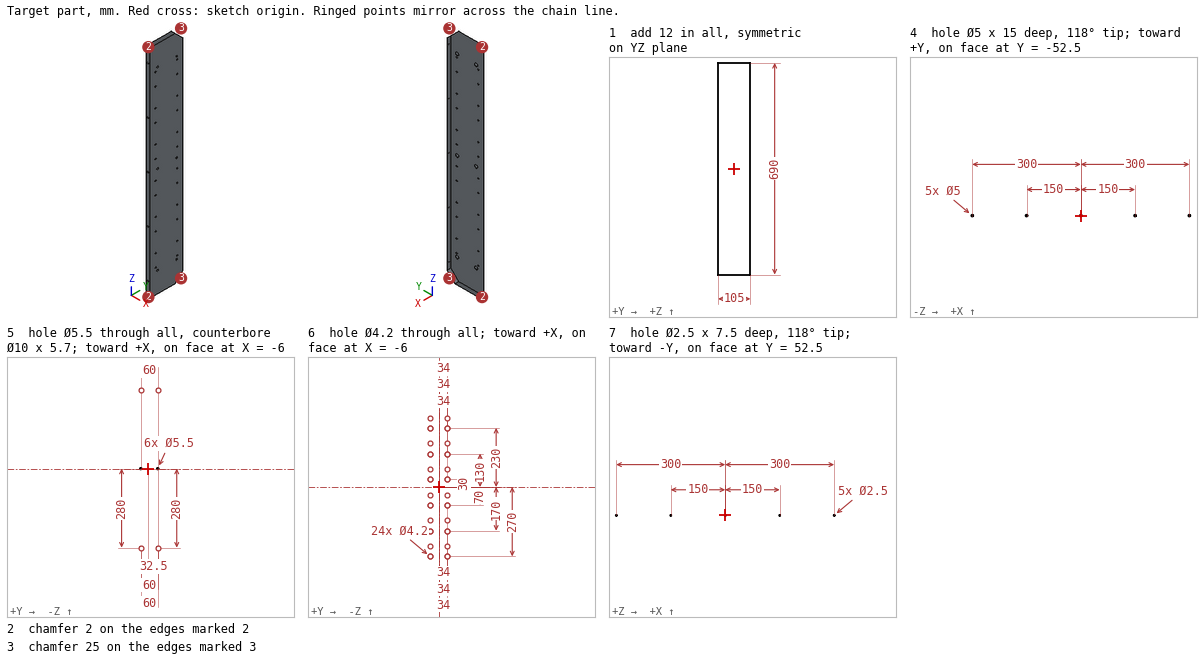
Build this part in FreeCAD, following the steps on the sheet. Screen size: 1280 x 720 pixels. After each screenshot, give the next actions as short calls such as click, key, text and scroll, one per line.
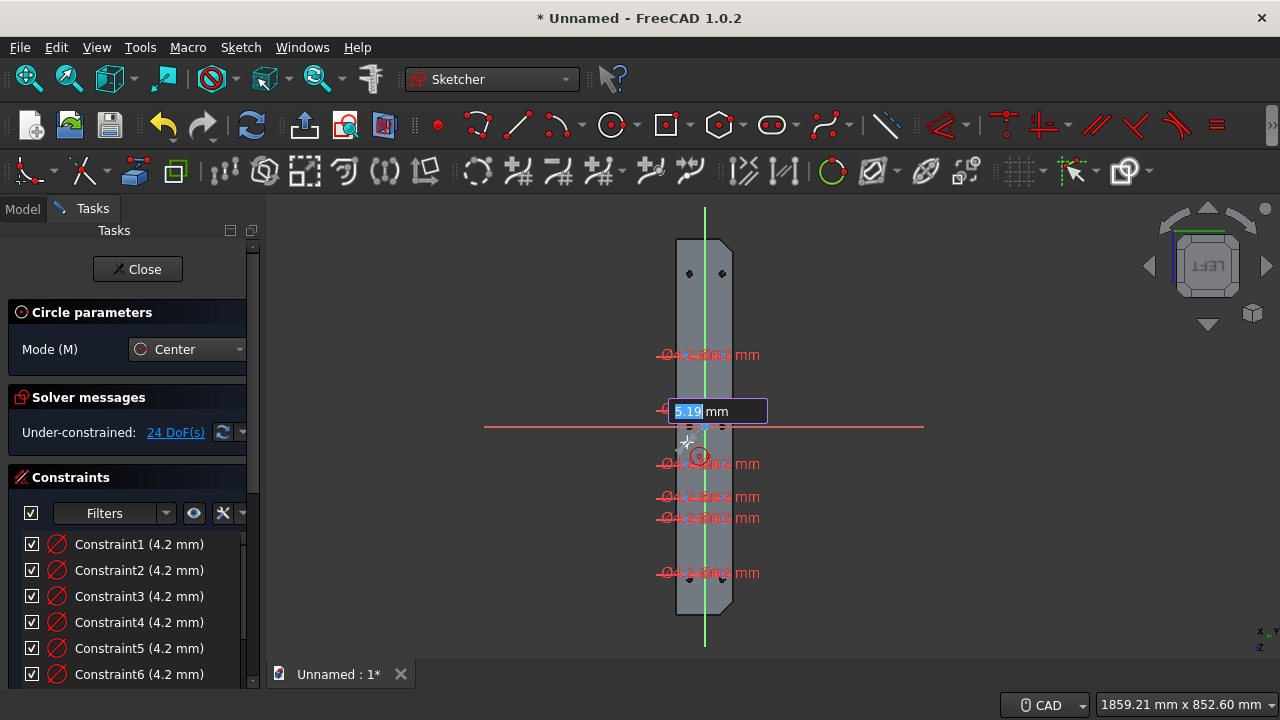
text(4.2)
key(Return)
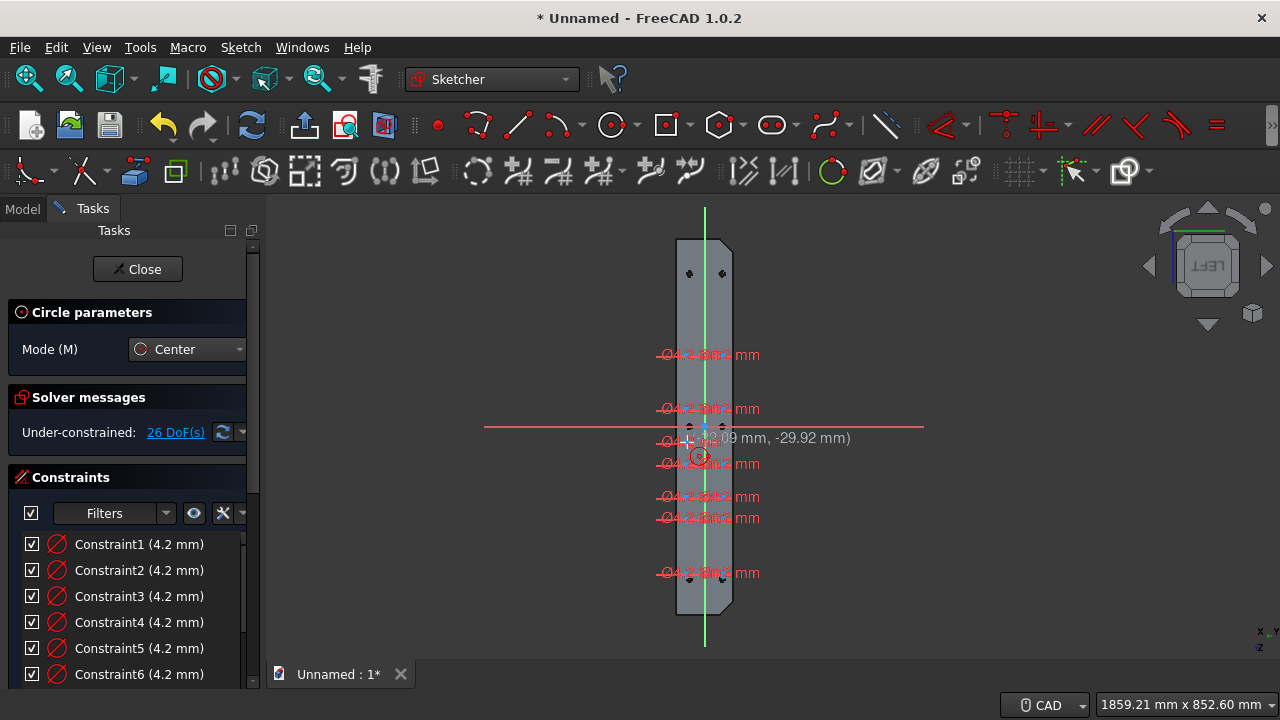
scroll(723, 443, up, 15)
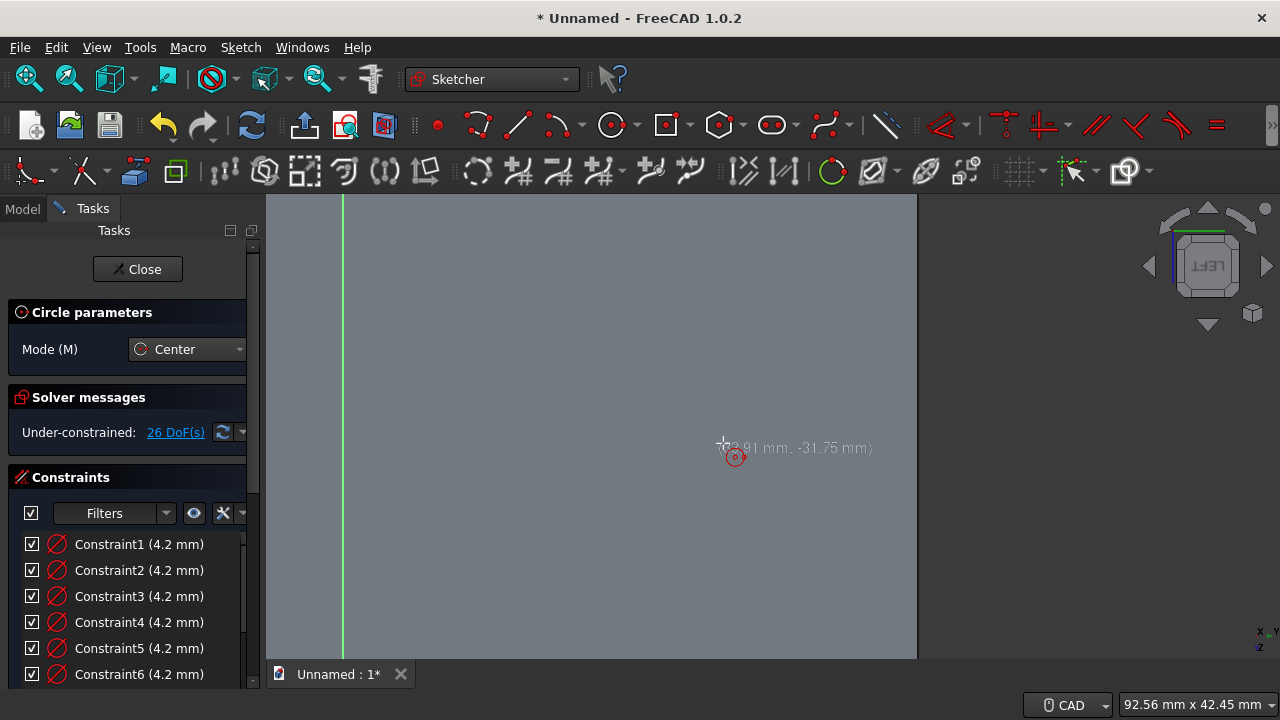
scroll(723, 443, down, 15)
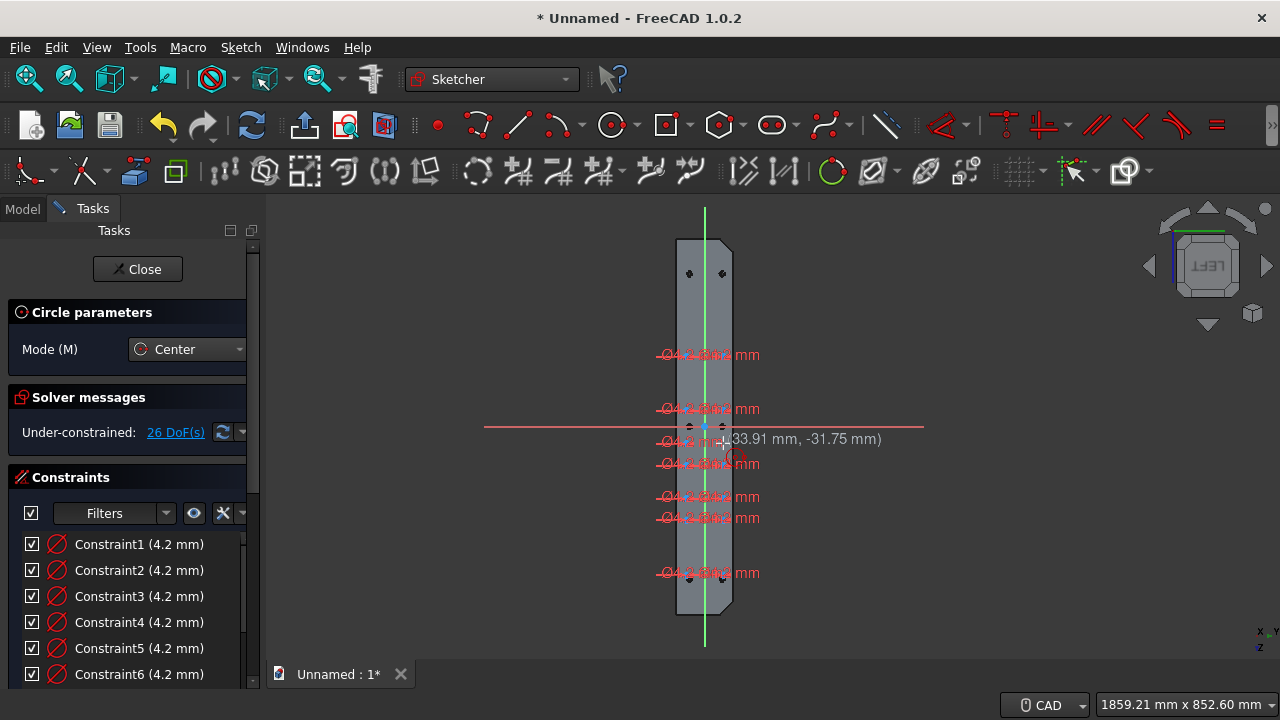
click(723, 443)
move(724, 442)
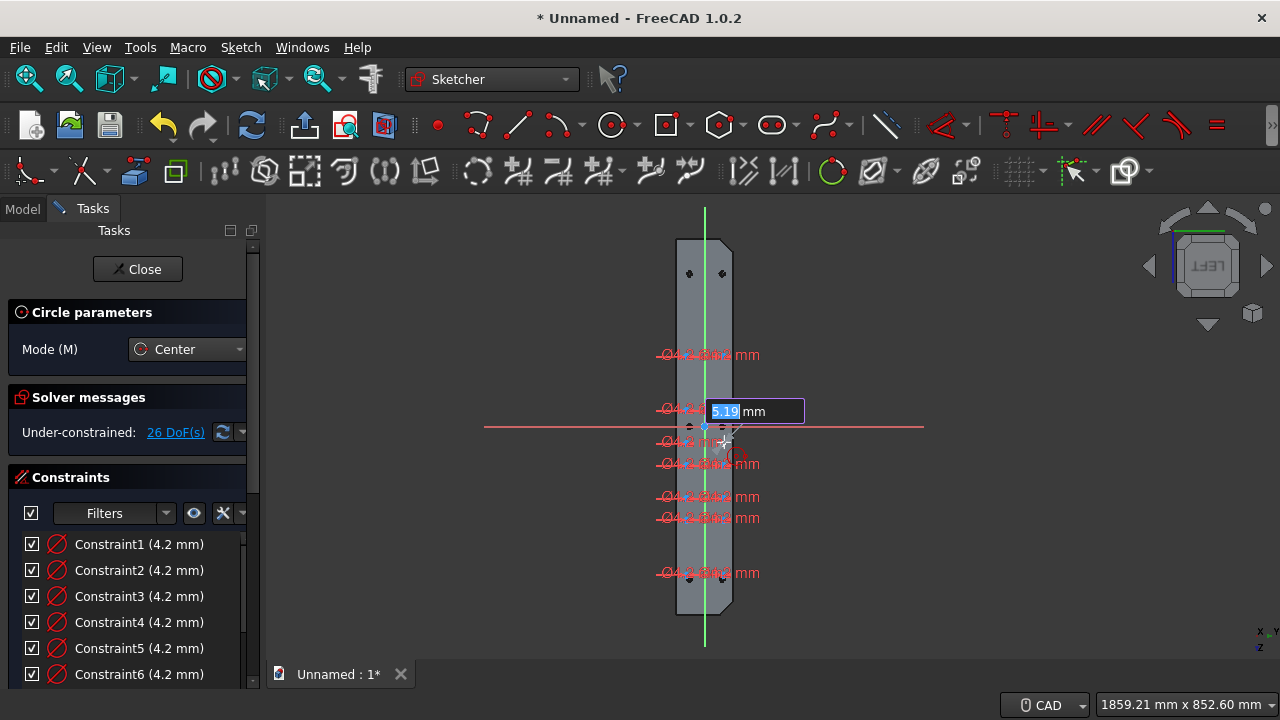
text(4.2)
key(Return)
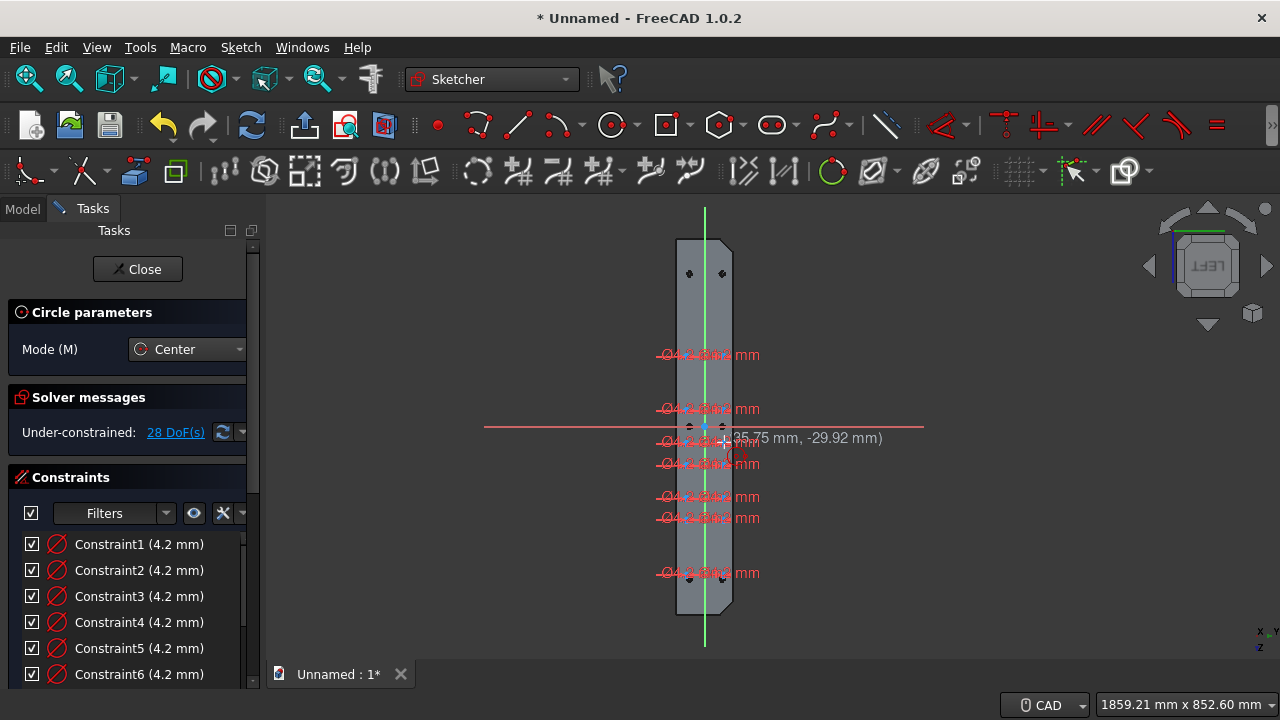
scroll(686, 389, up, 15)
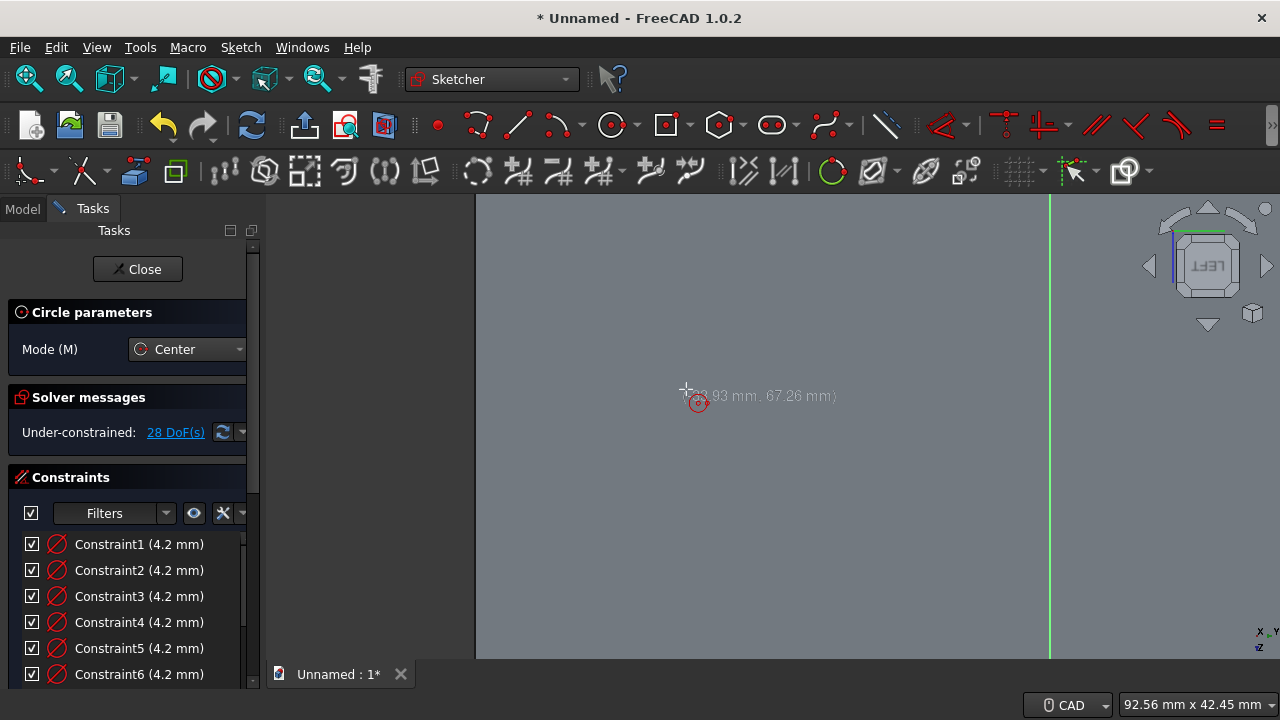
scroll(686, 389, down, 15)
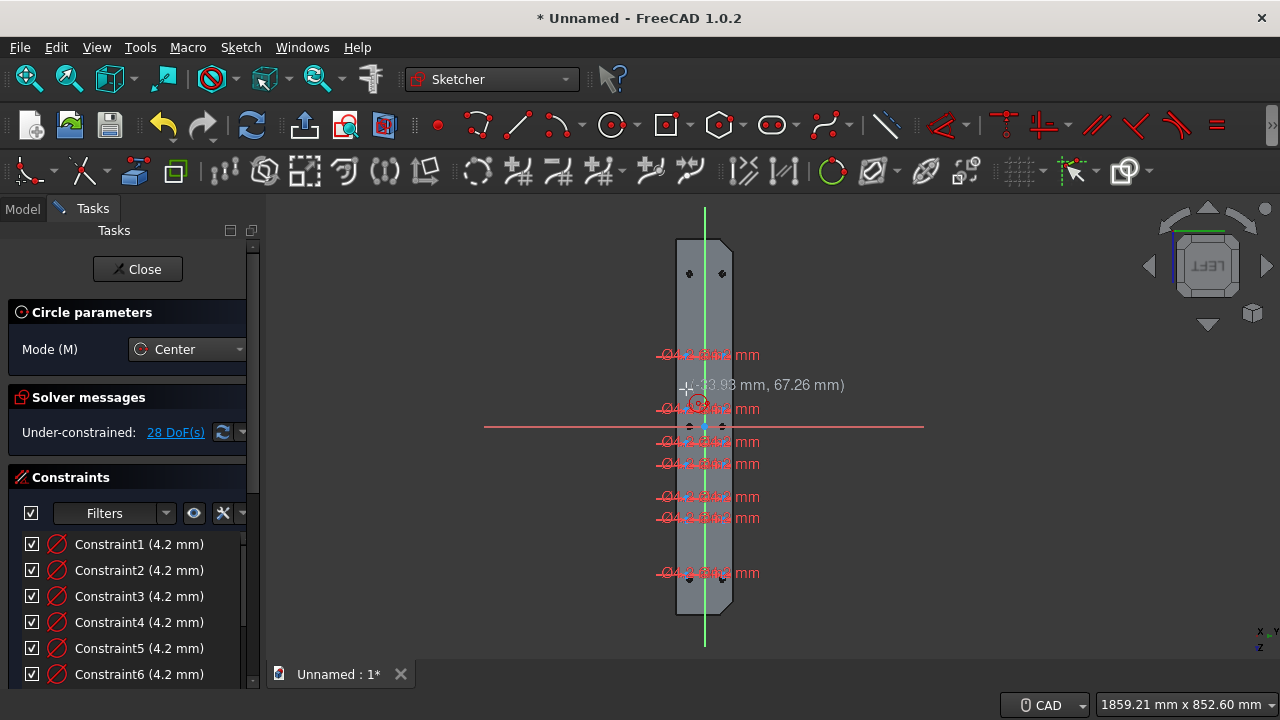
click(686, 389)
move(687, 388)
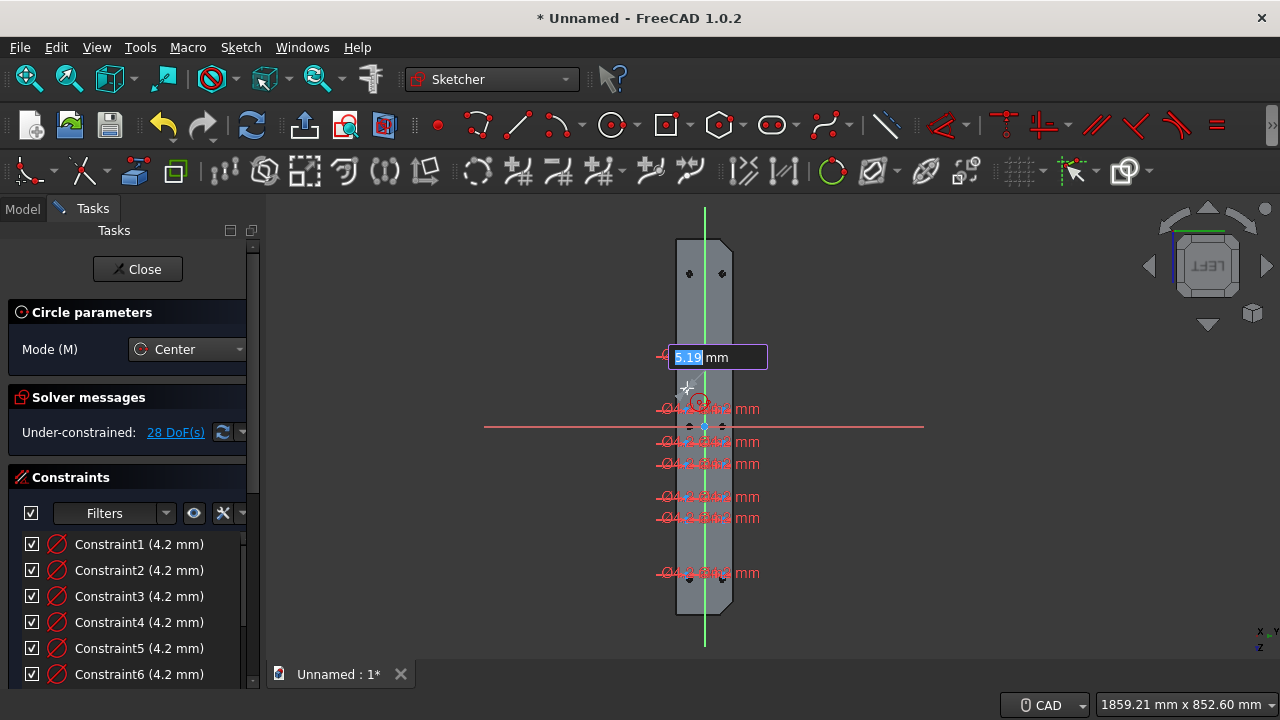
text(4.2)
key(Return)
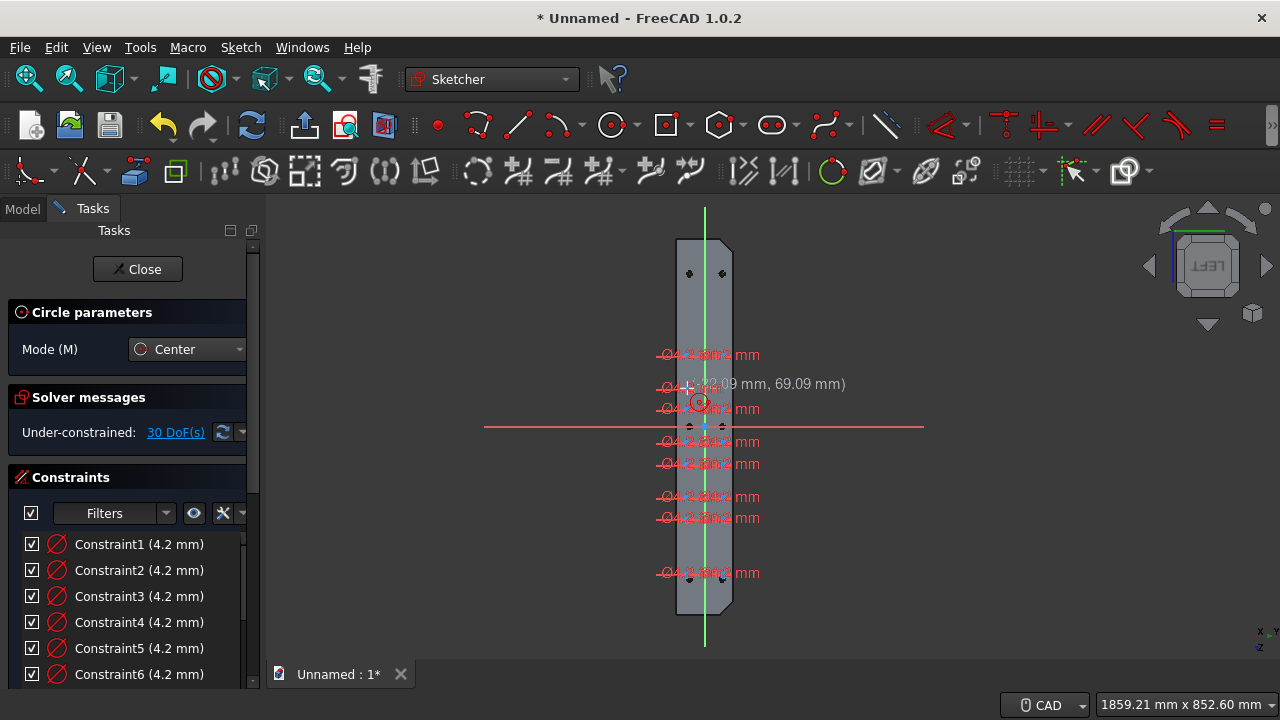
scroll(723, 389, up, 15)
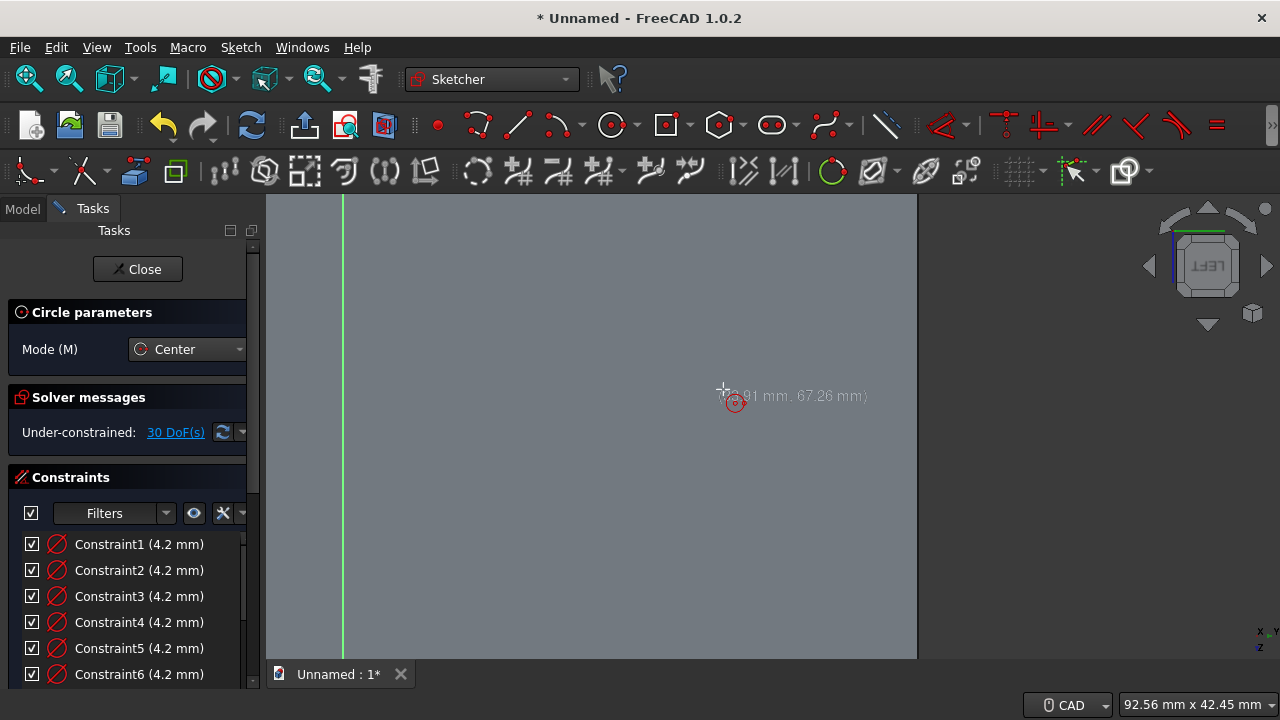
scroll(723, 389, down, 15)